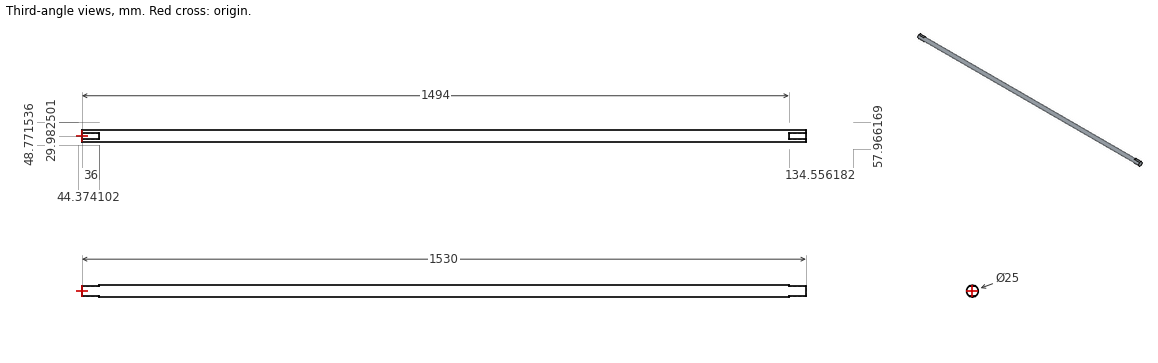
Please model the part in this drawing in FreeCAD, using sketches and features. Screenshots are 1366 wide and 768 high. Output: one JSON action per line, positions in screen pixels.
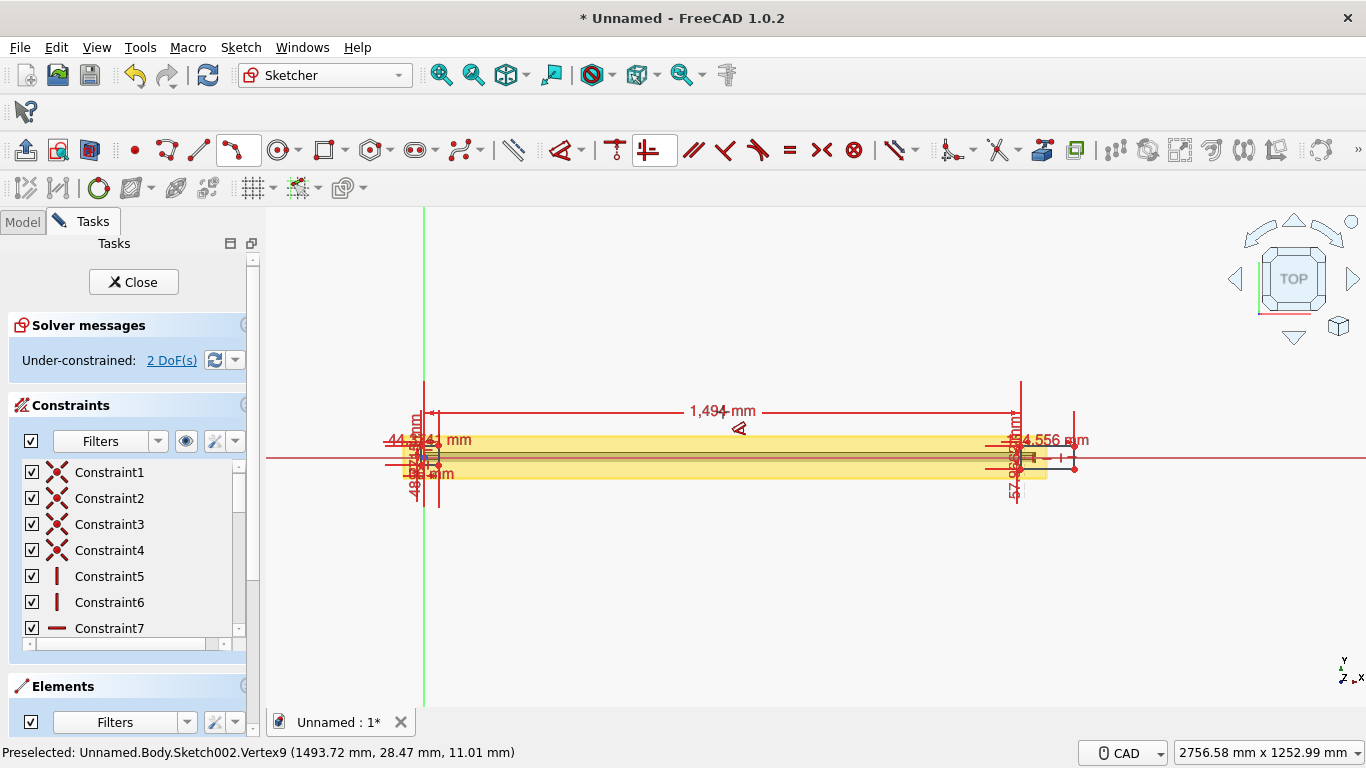
{"action": "scroll", "coordinate": [421, 446], "scroll_direction": "up", "scroll_amount": 6}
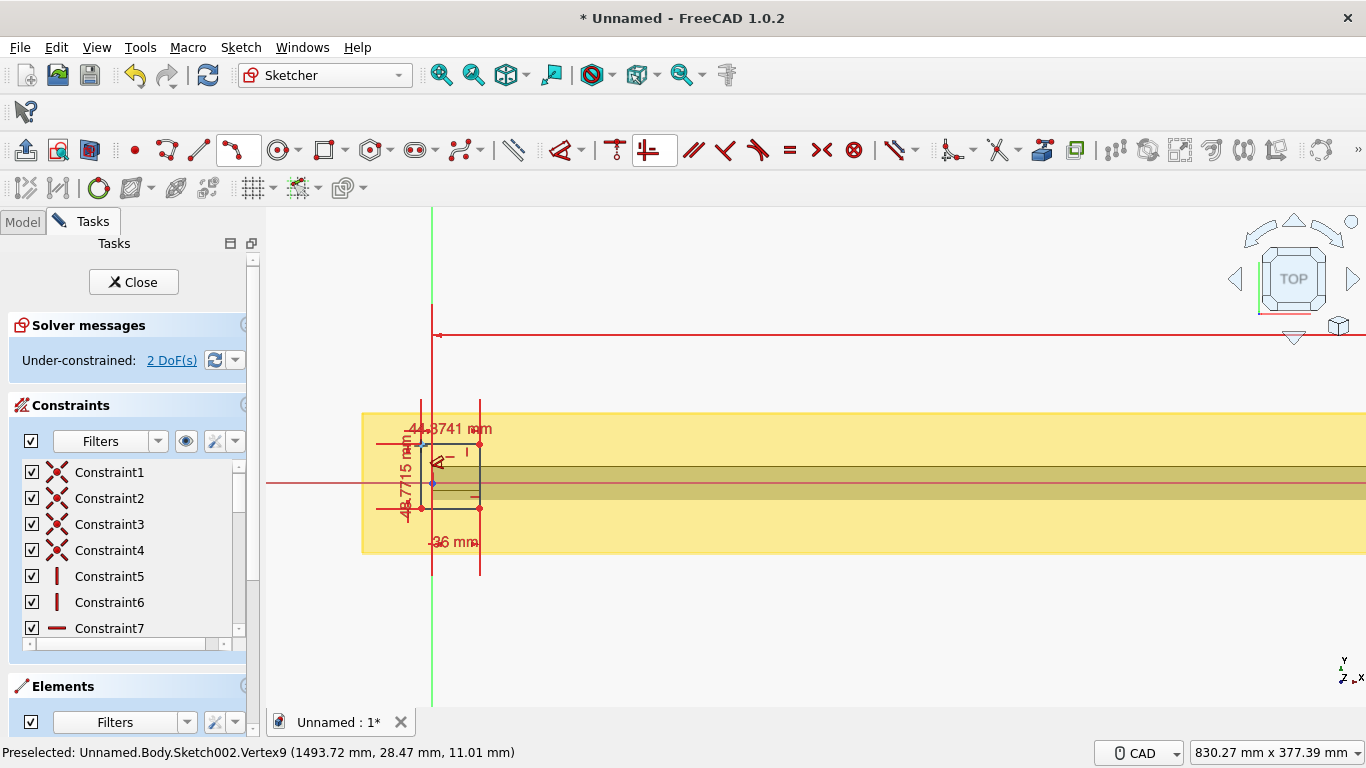
{"action": "left_click", "coordinate": [421, 444]}
{"action": "left_click", "coordinate": [387, 464]}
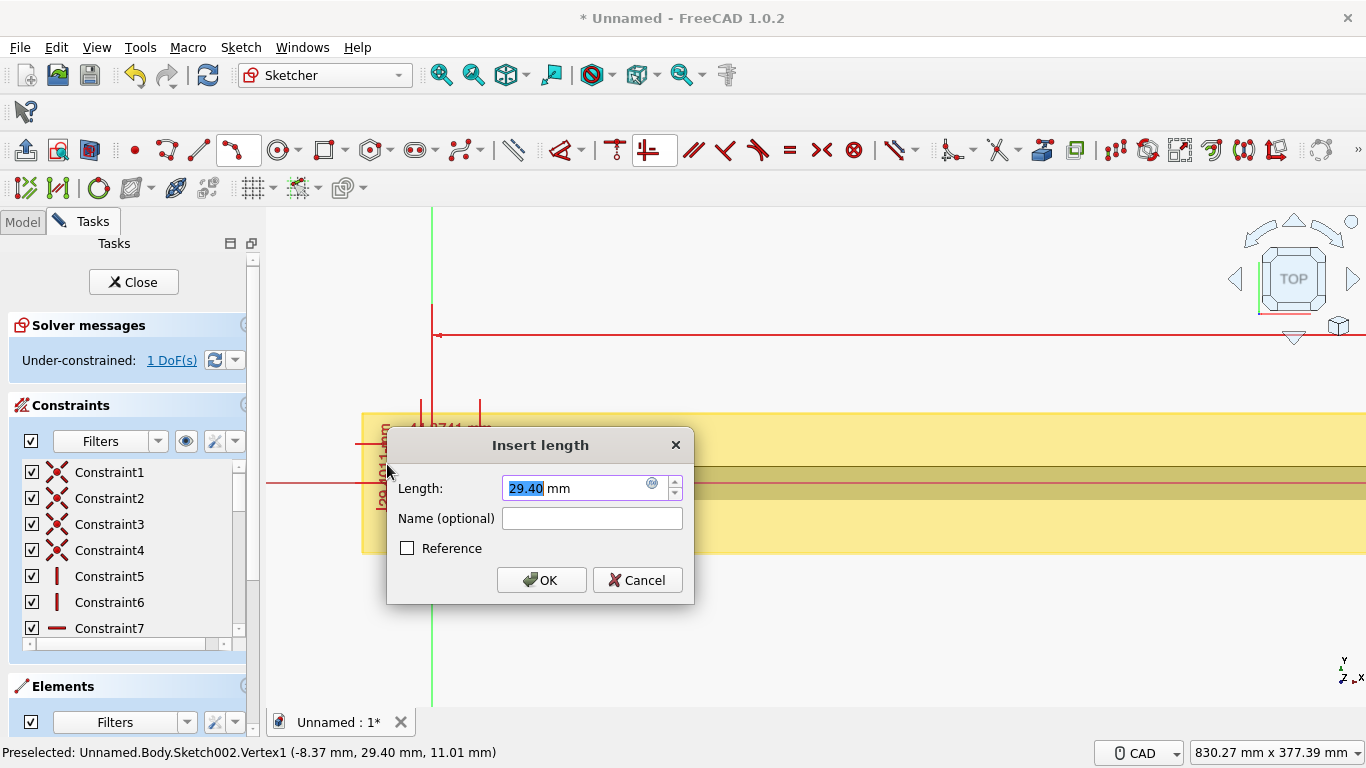
{"action": "type", "text": "29.982501"}
{"action": "key", "text": "Return"}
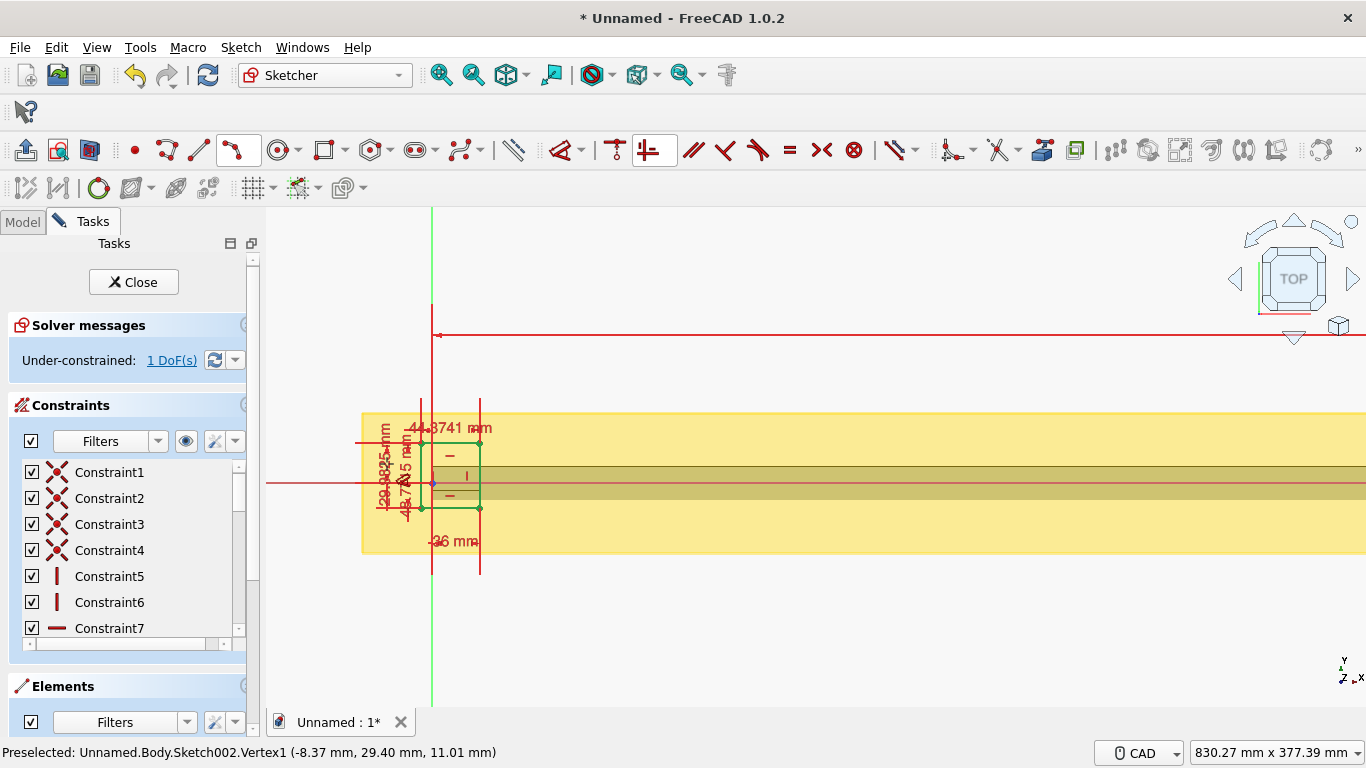
{"action": "scroll", "coordinate": [421, 446], "scroll_direction": "down", "scroll_amount": 6}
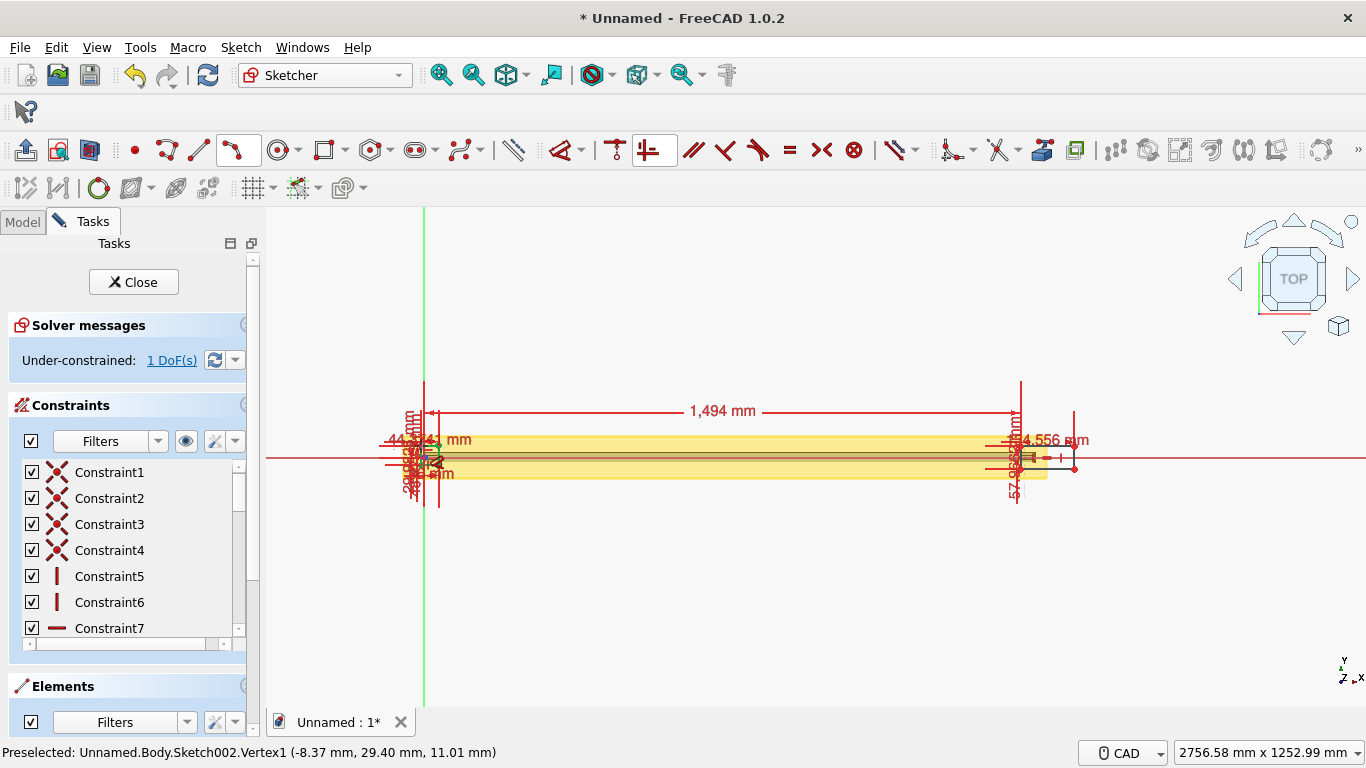
{"action": "scroll", "coordinate": [1021, 446], "scroll_direction": "up", "scroll_amount": 6}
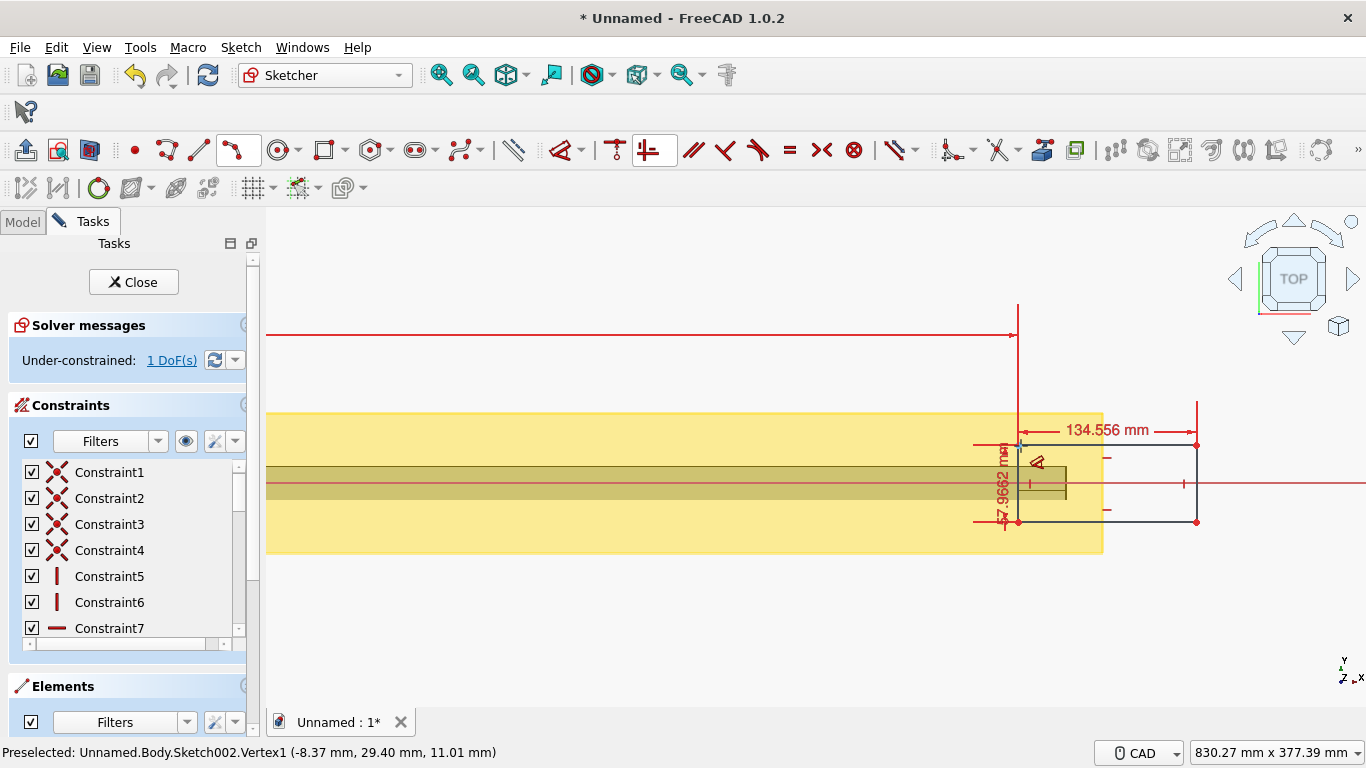
{"action": "left_click", "coordinate": [1018, 445]}
{"action": "left_click", "coordinate": [1052, 464]}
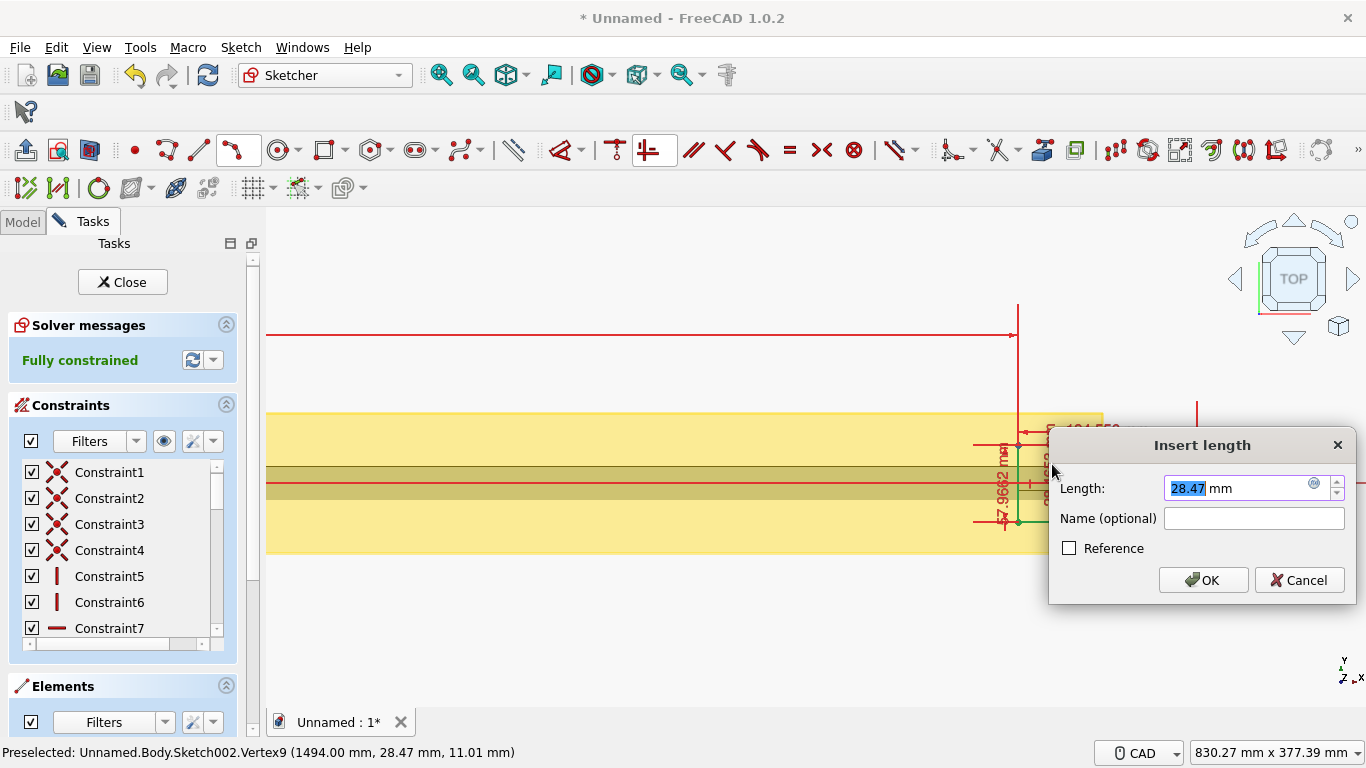
{"action": "type", "text": "29.982501"}
{"action": "key", "text": "Return"}
{"action": "key", "text": "Escape"}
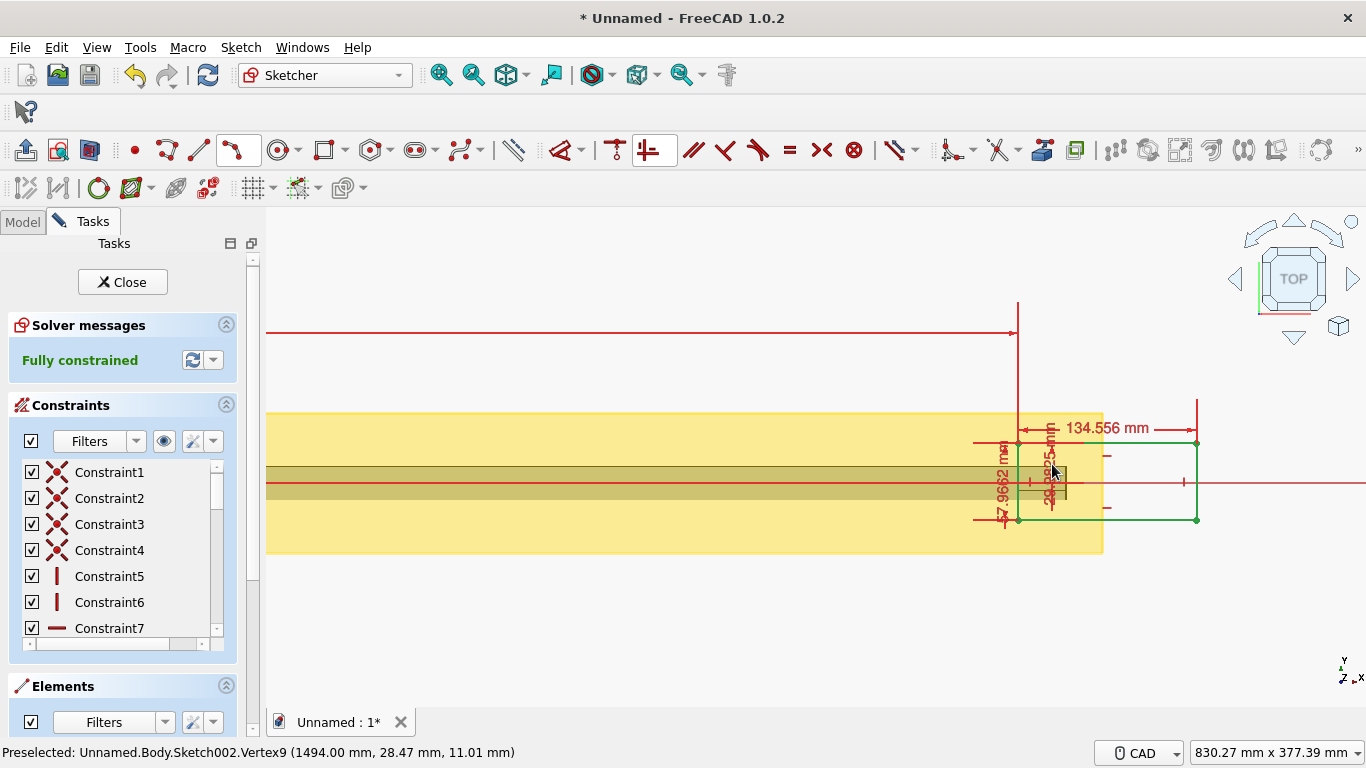
{"action": "left_click", "coordinate": [123, 282]}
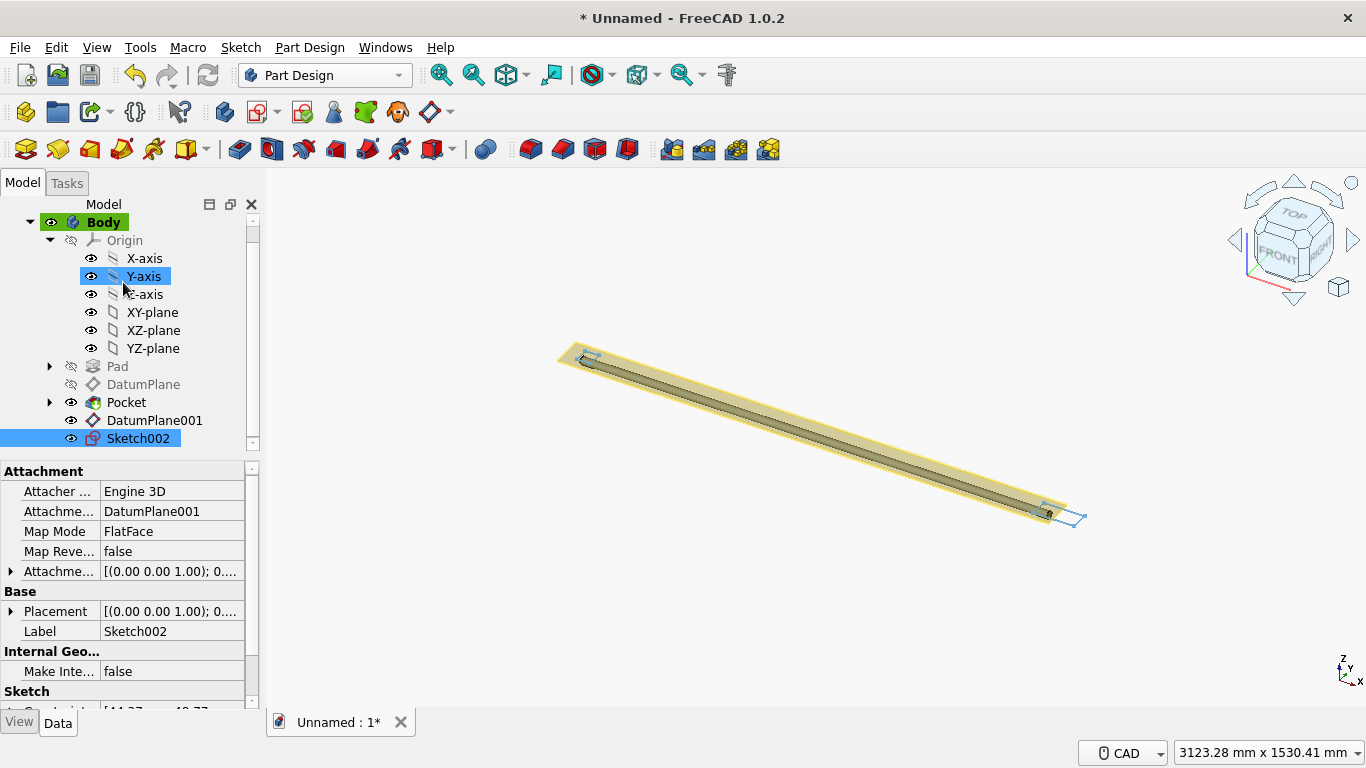
{"action": "left_click", "coordinate": [240, 150]}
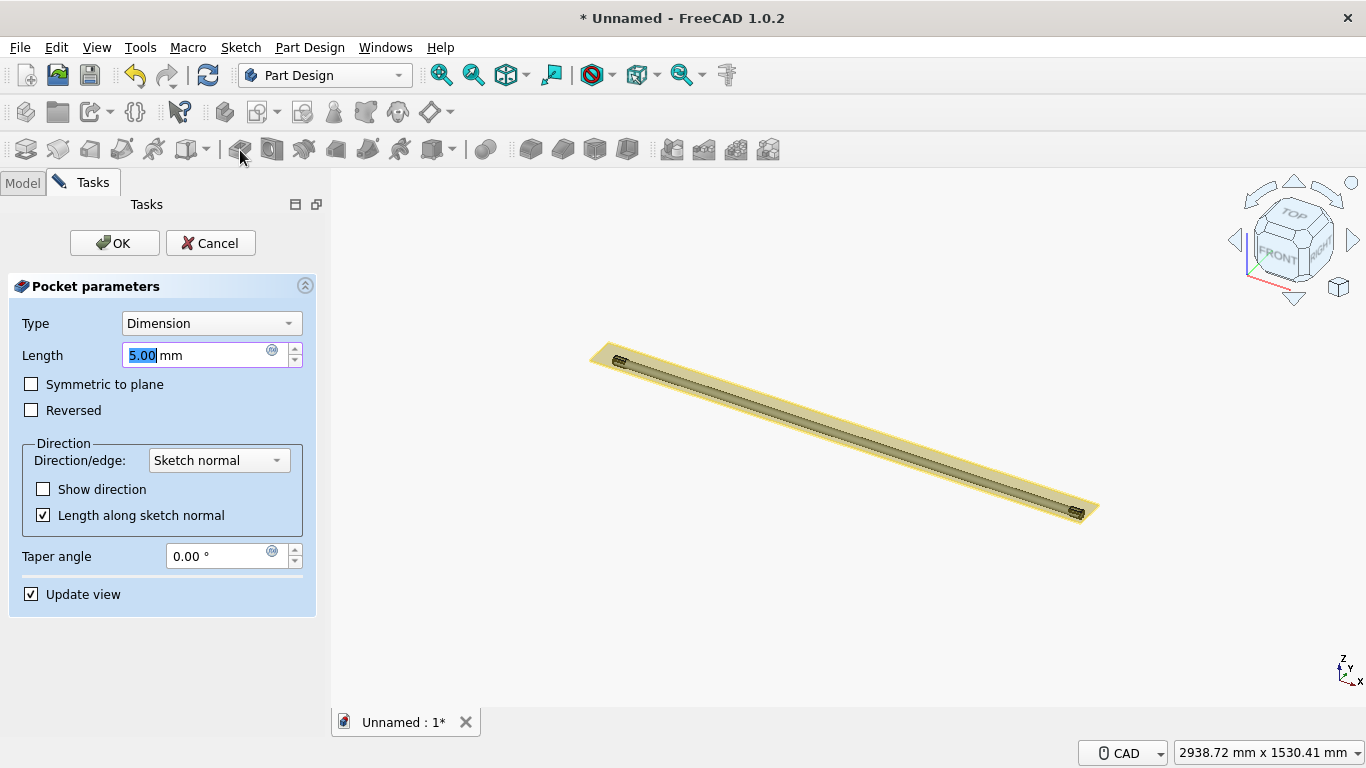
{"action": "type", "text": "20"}
{"action": "key", "text": "Tab"}